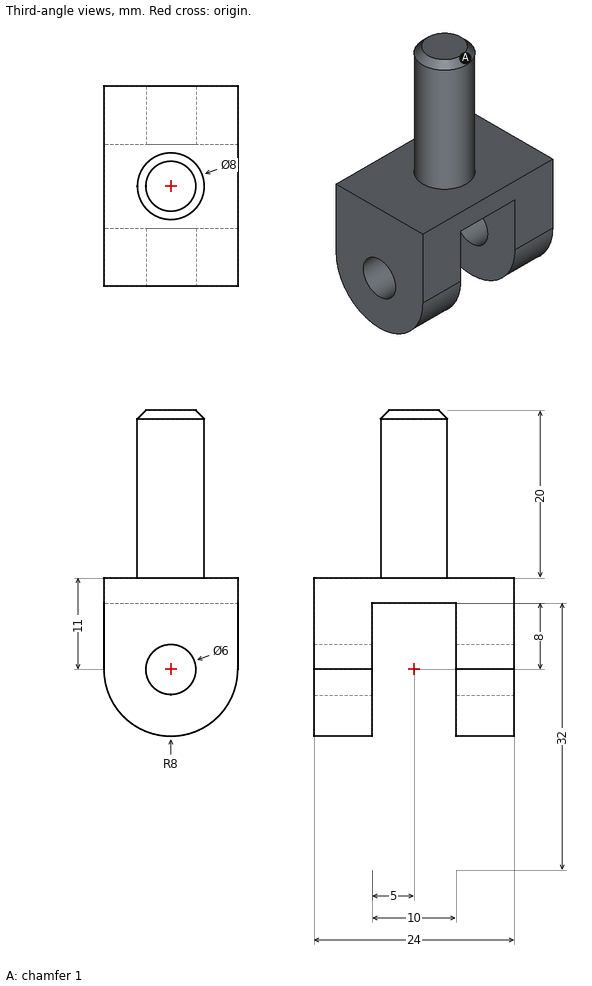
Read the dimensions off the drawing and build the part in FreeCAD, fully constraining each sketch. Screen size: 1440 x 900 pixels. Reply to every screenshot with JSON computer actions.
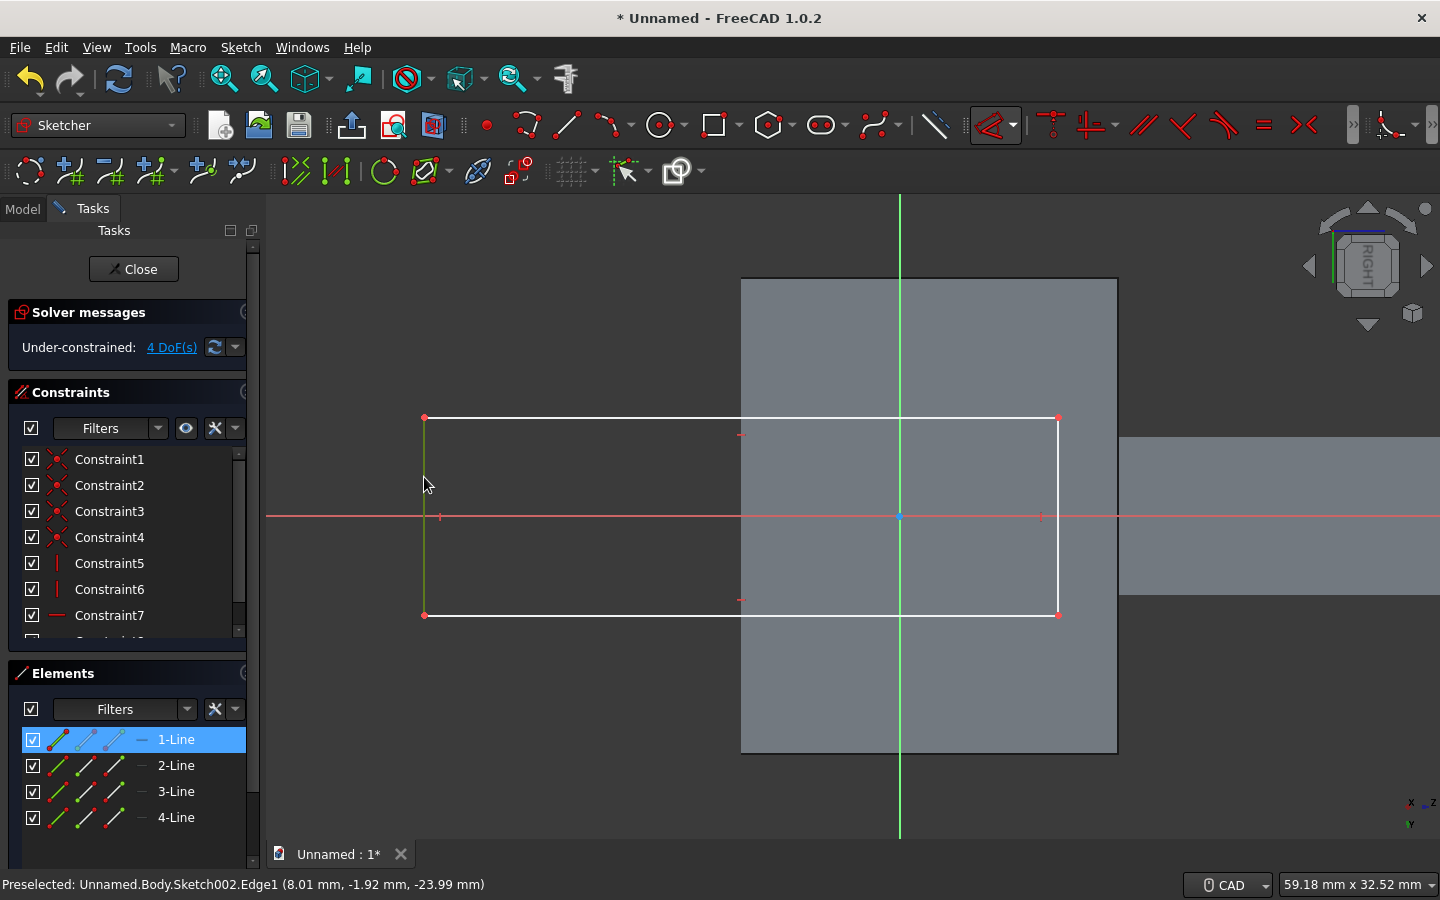
{"action": "left_click", "coordinate": [1016, 126]}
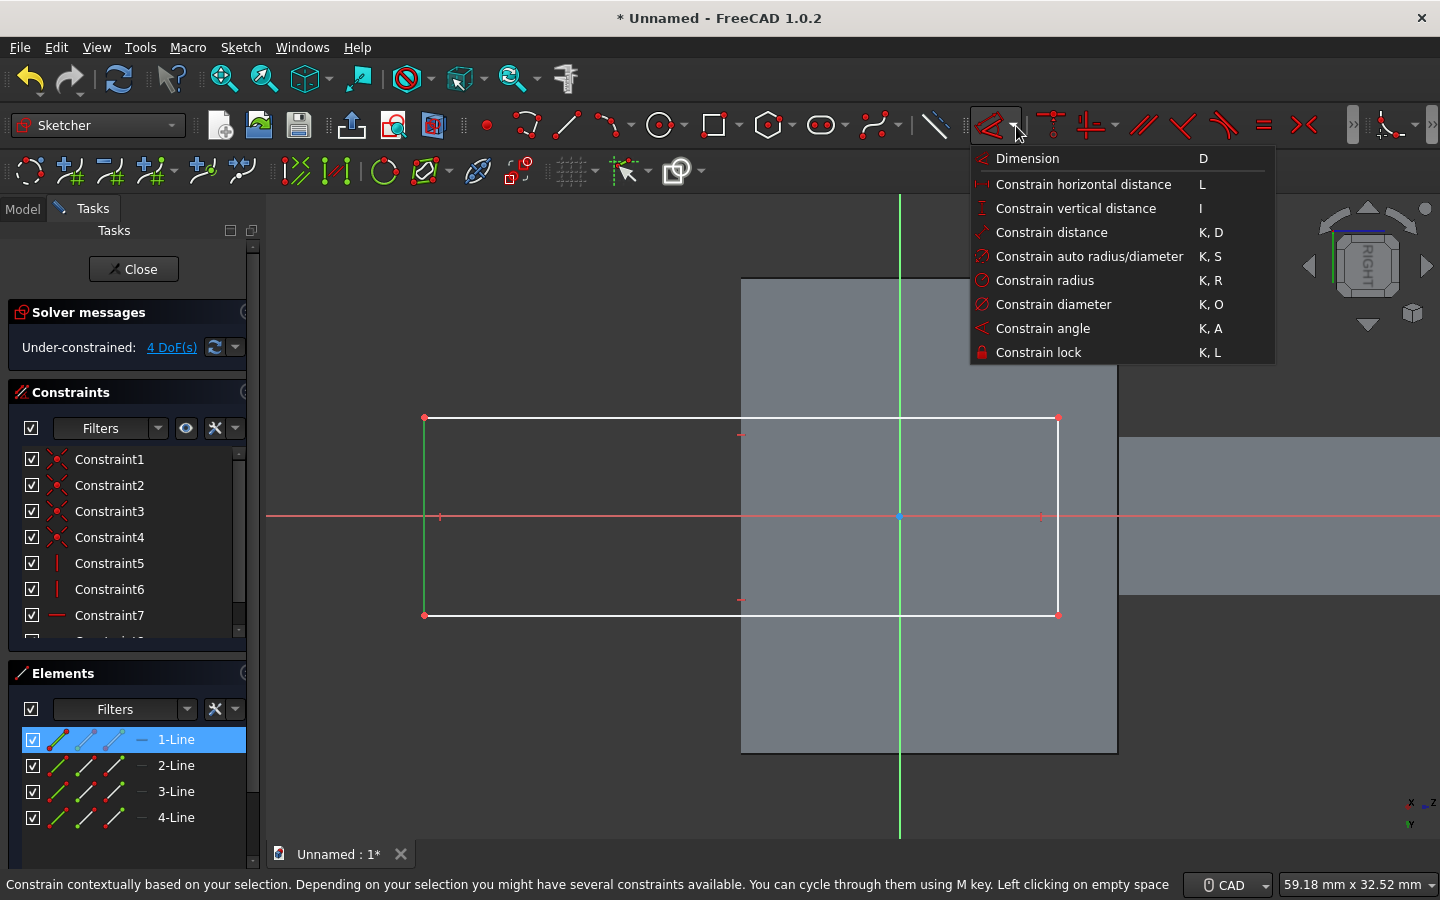
{"action": "left_click", "coordinate": [1123, 208]}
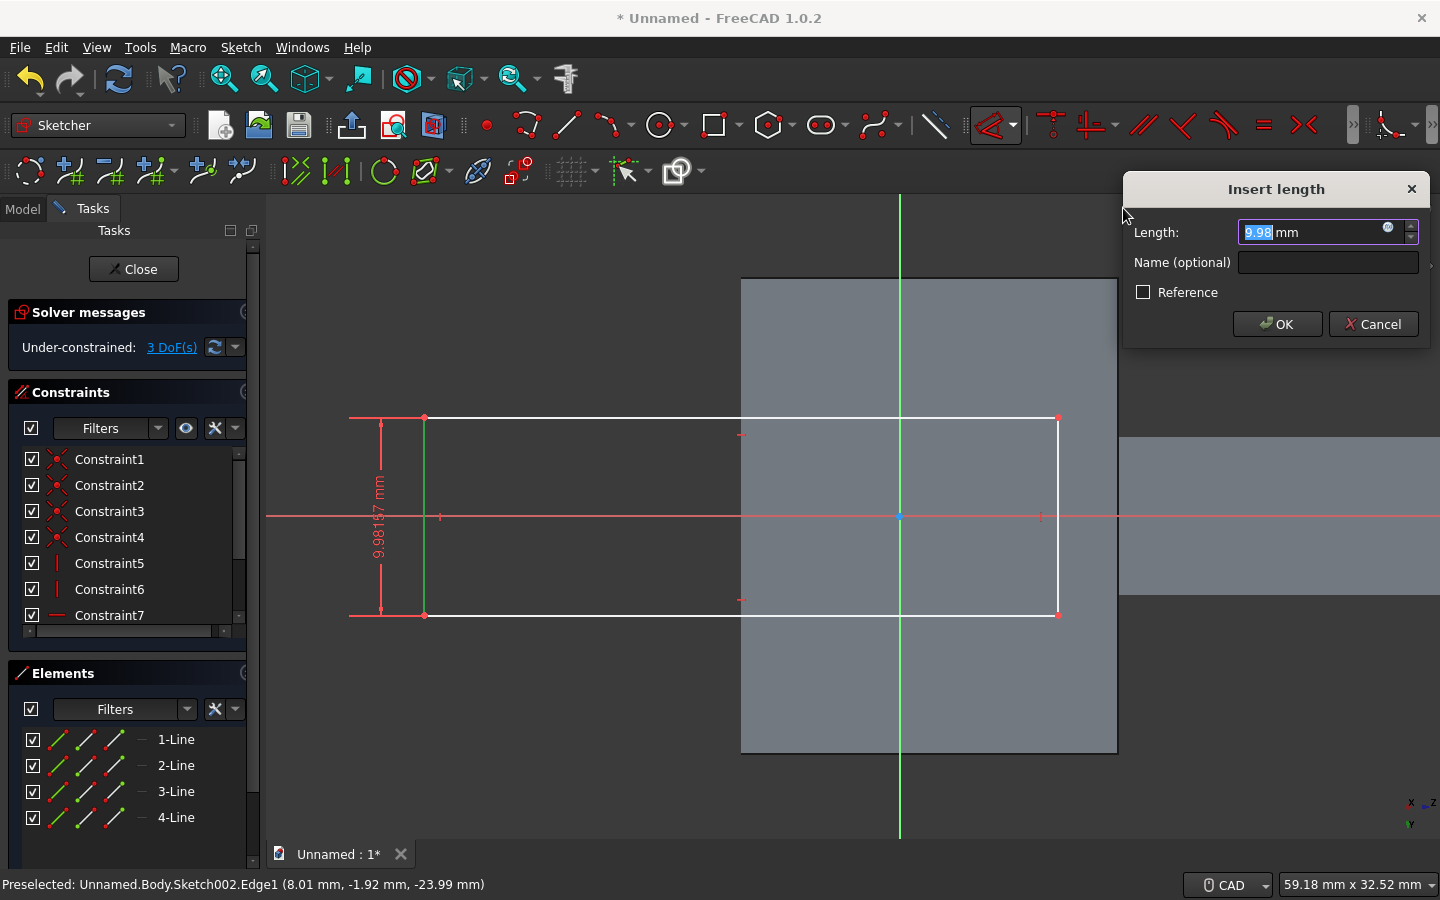
{"action": "type", "text": "10"}
{"action": "key", "text": "Return"}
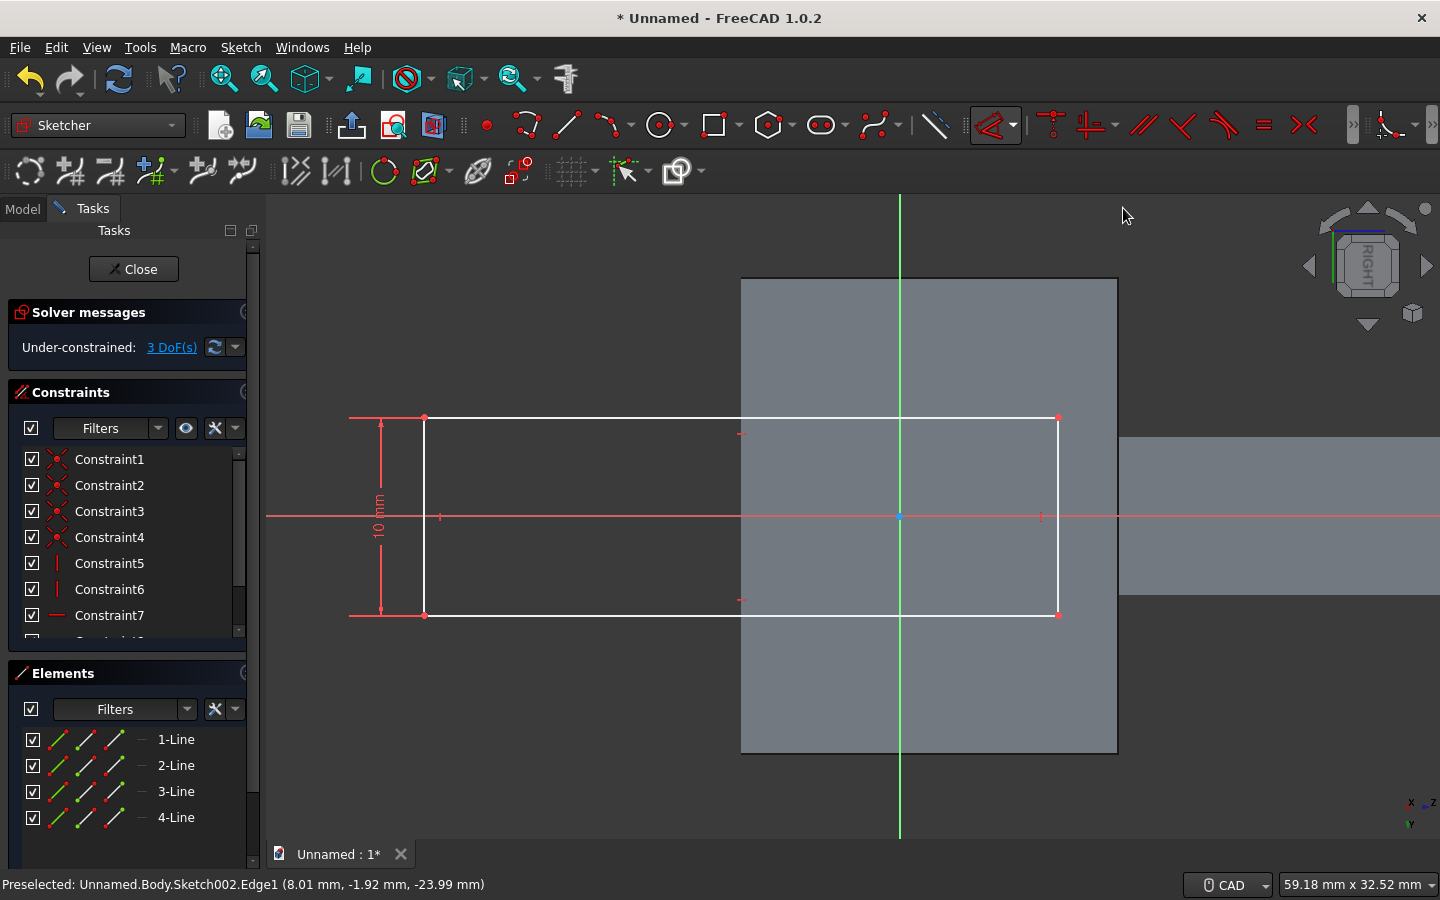
{"action": "left_click", "coordinate": [614, 616]}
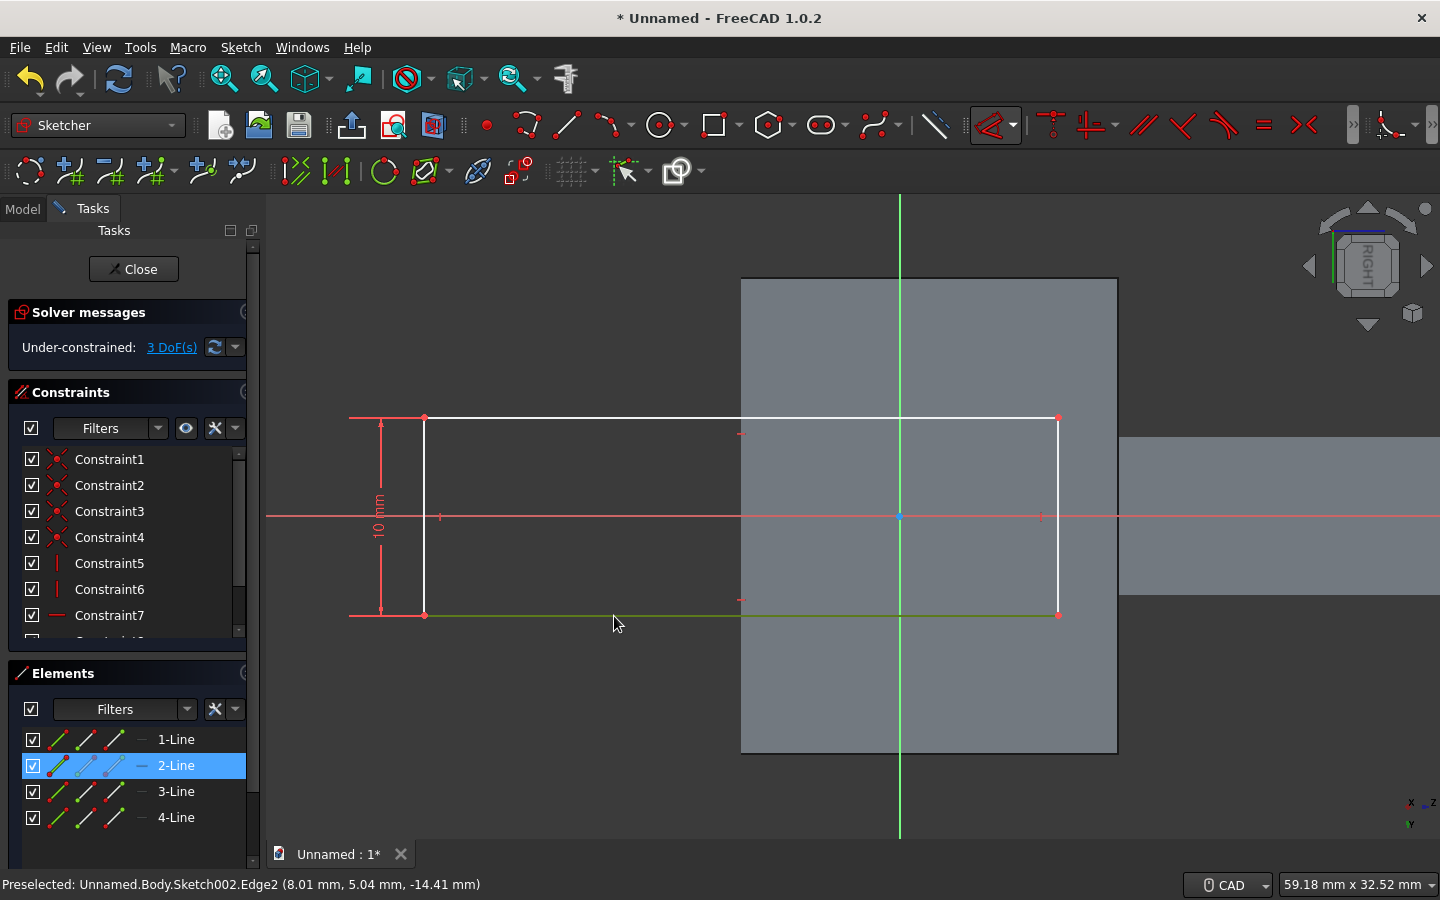
{"action": "left_click", "coordinate": [1016, 126]}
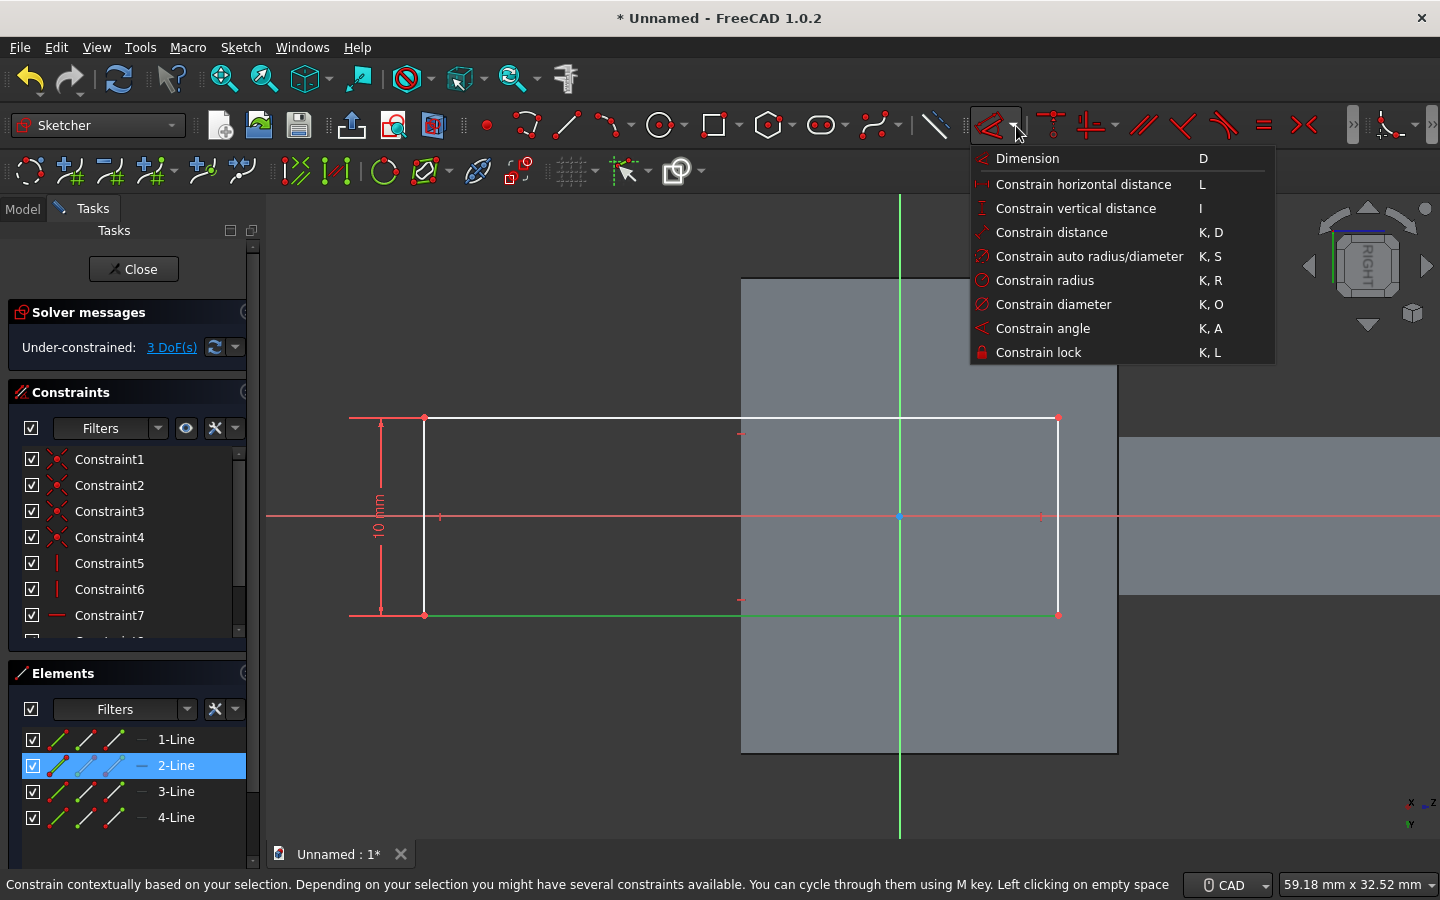
{"action": "left_click", "coordinate": [1123, 184]}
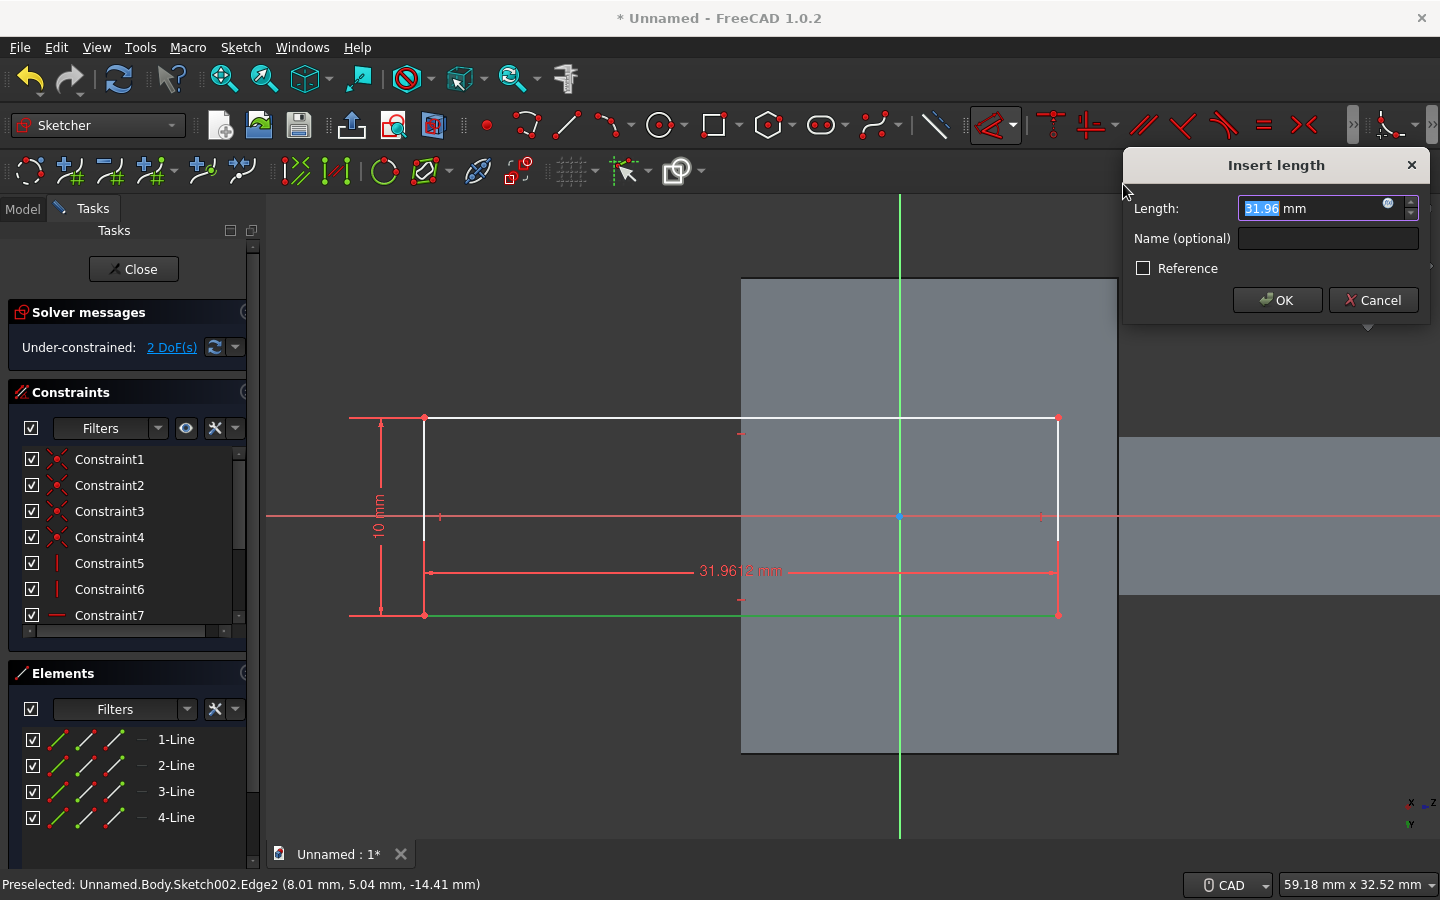
{"action": "type", "text": "32"}
{"action": "key", "text": "Return"}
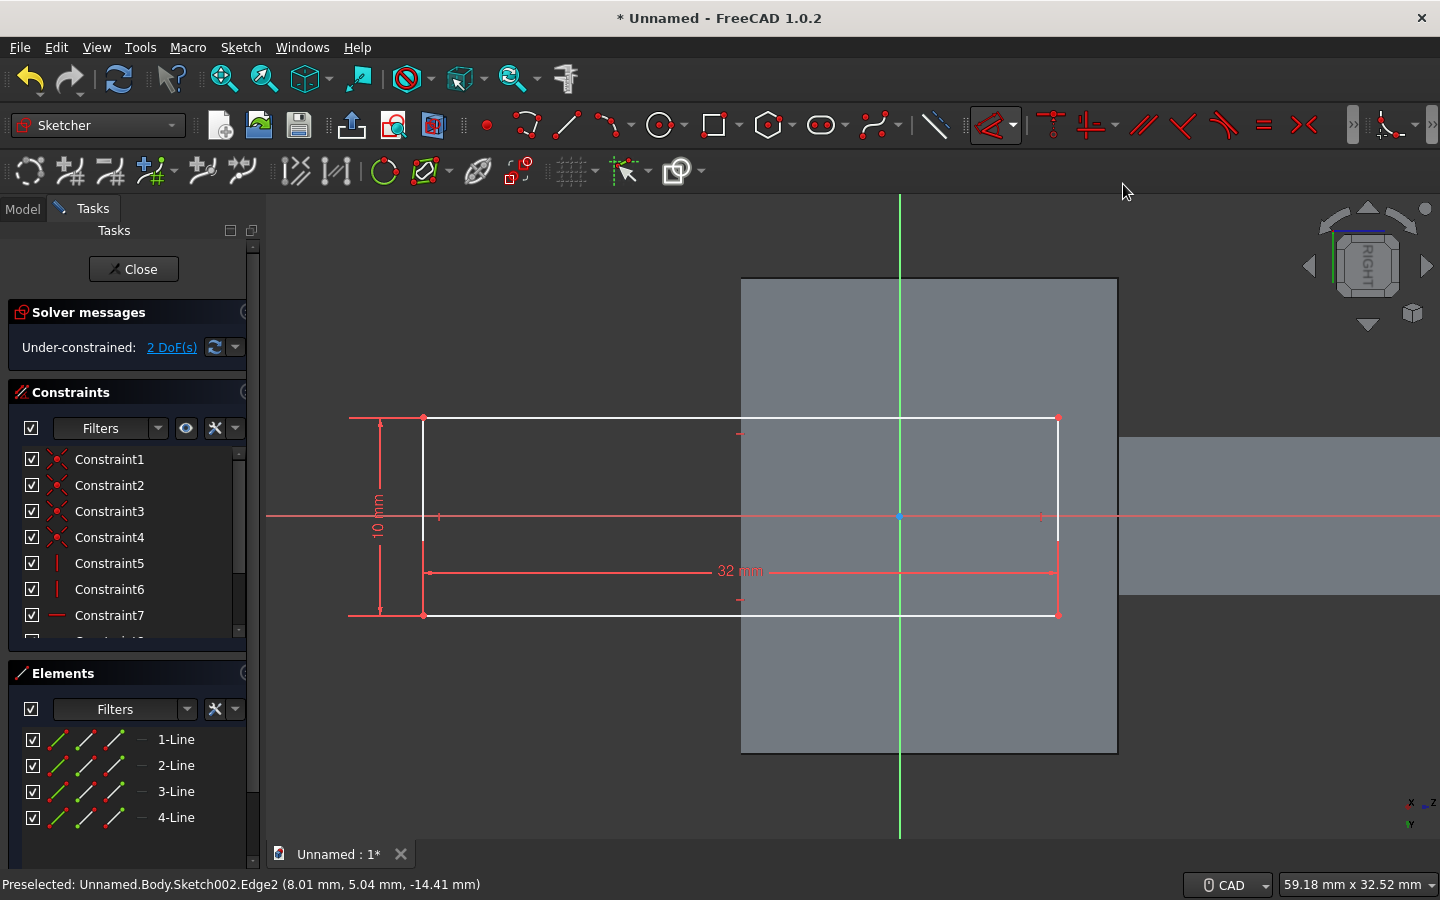
{"action": "left_click", "coordinate": [423, 418]}